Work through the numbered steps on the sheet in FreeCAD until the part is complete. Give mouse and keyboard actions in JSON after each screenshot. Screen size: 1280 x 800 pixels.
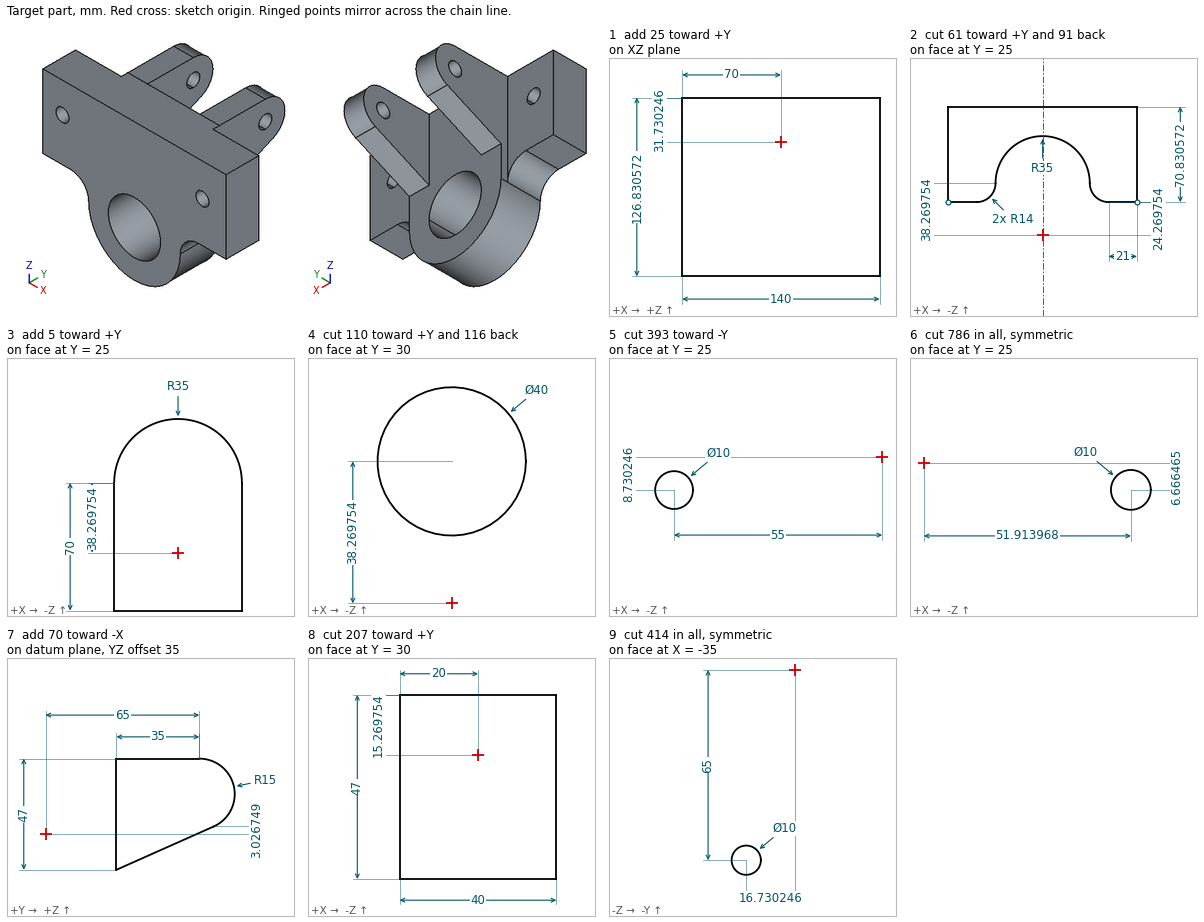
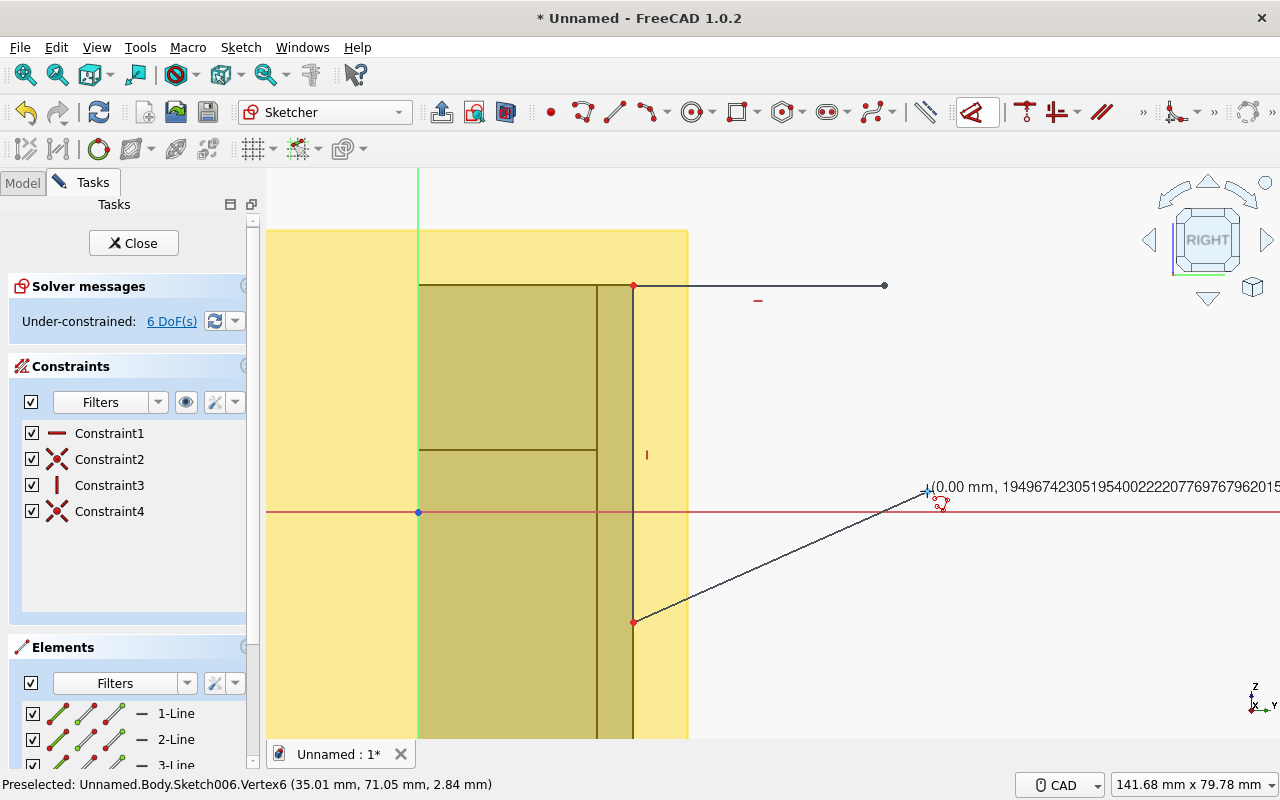
{"action": "left_click", "coordinate": [648, 112]}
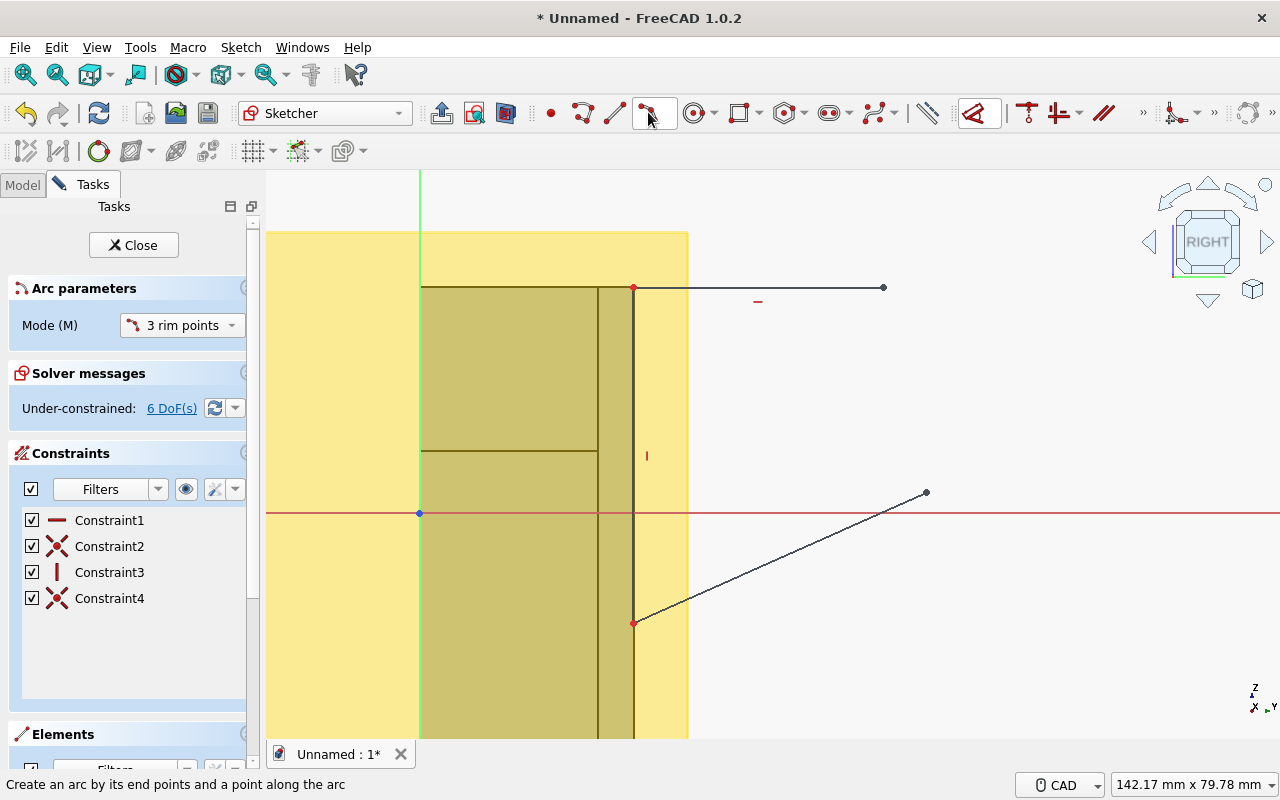
{"action": "left_click", "coordinate": [926, 493]}
{"action": "left_click", "coordinate": [884, 288]}
{"action": "left_click", "coordinate": [988, 372]}
{"action": "key", "text": "Escape"}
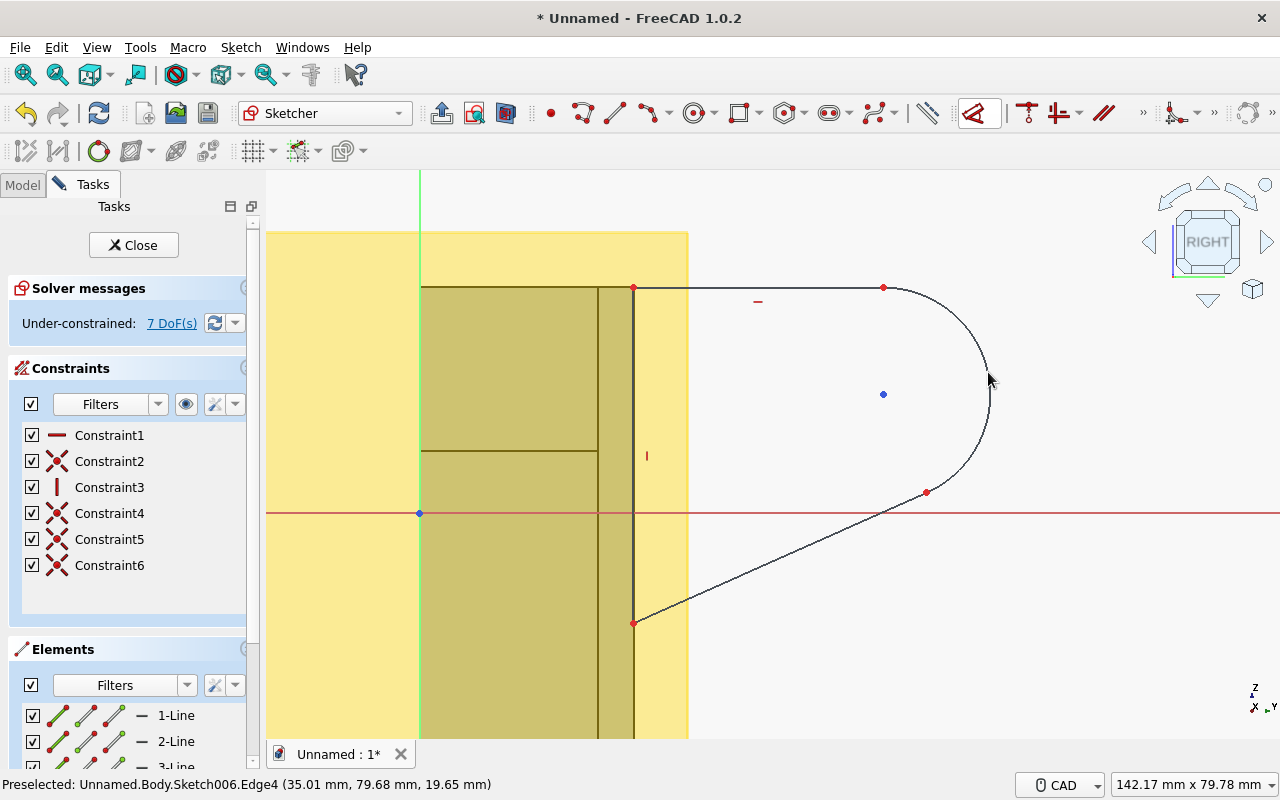
{"action": "left_click", "coordinate": [809, 288]}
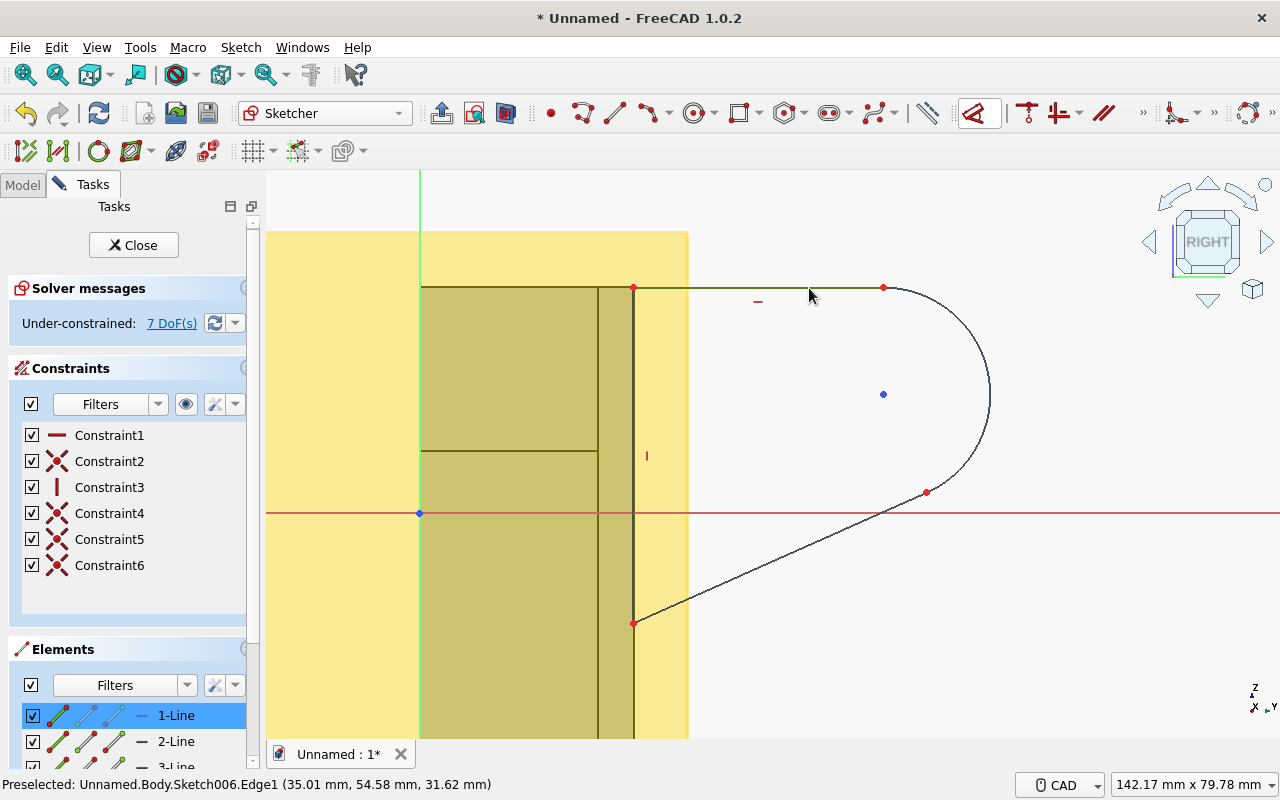
{"action": "left_click", "coordinate": [984, 430]}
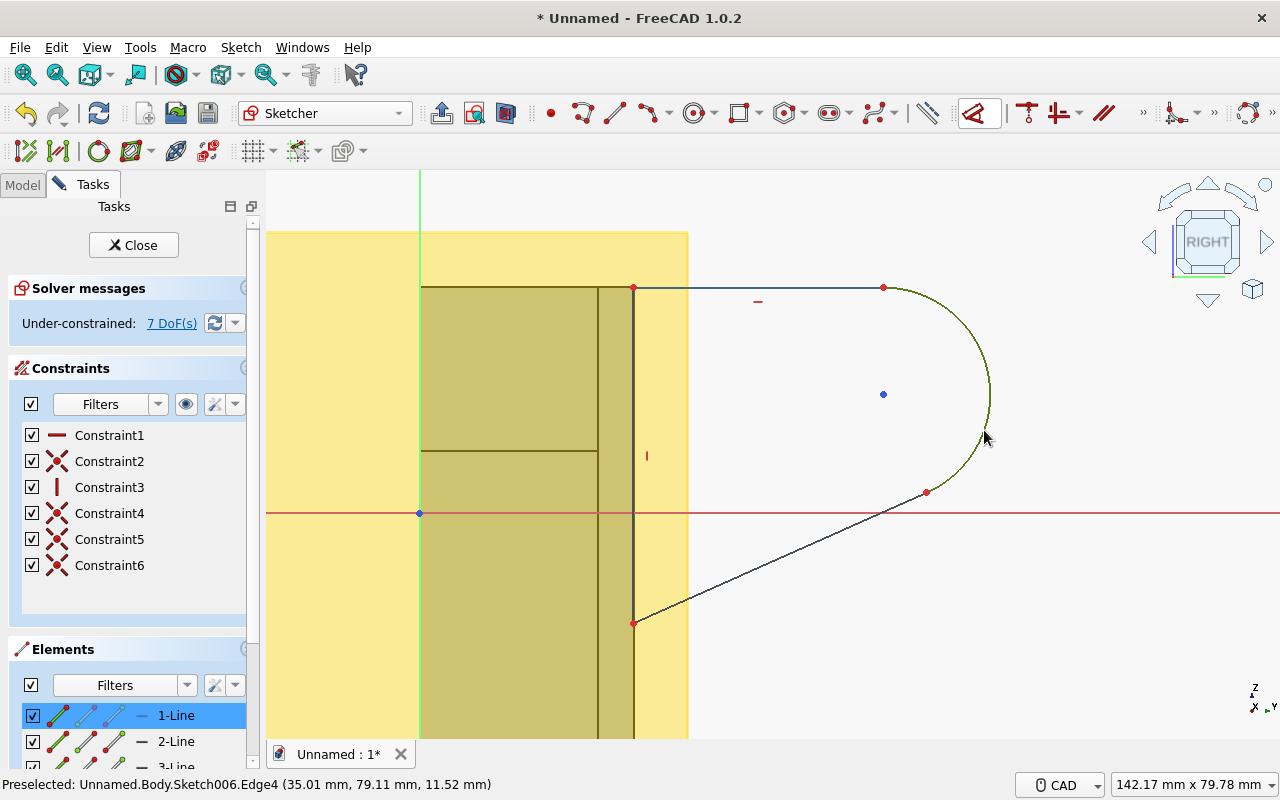
{"action": "key", "text": "t"}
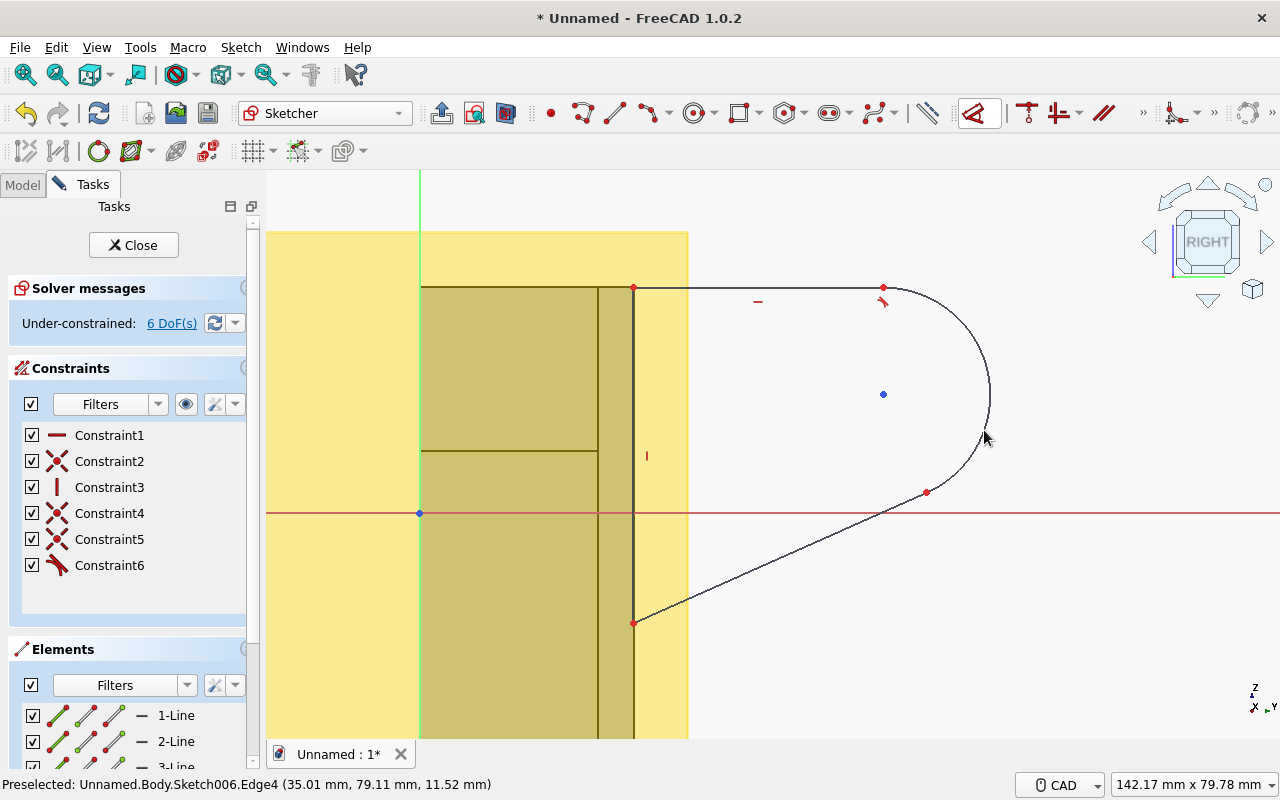
{"action": "left_click", "coordinate": [721, 584]}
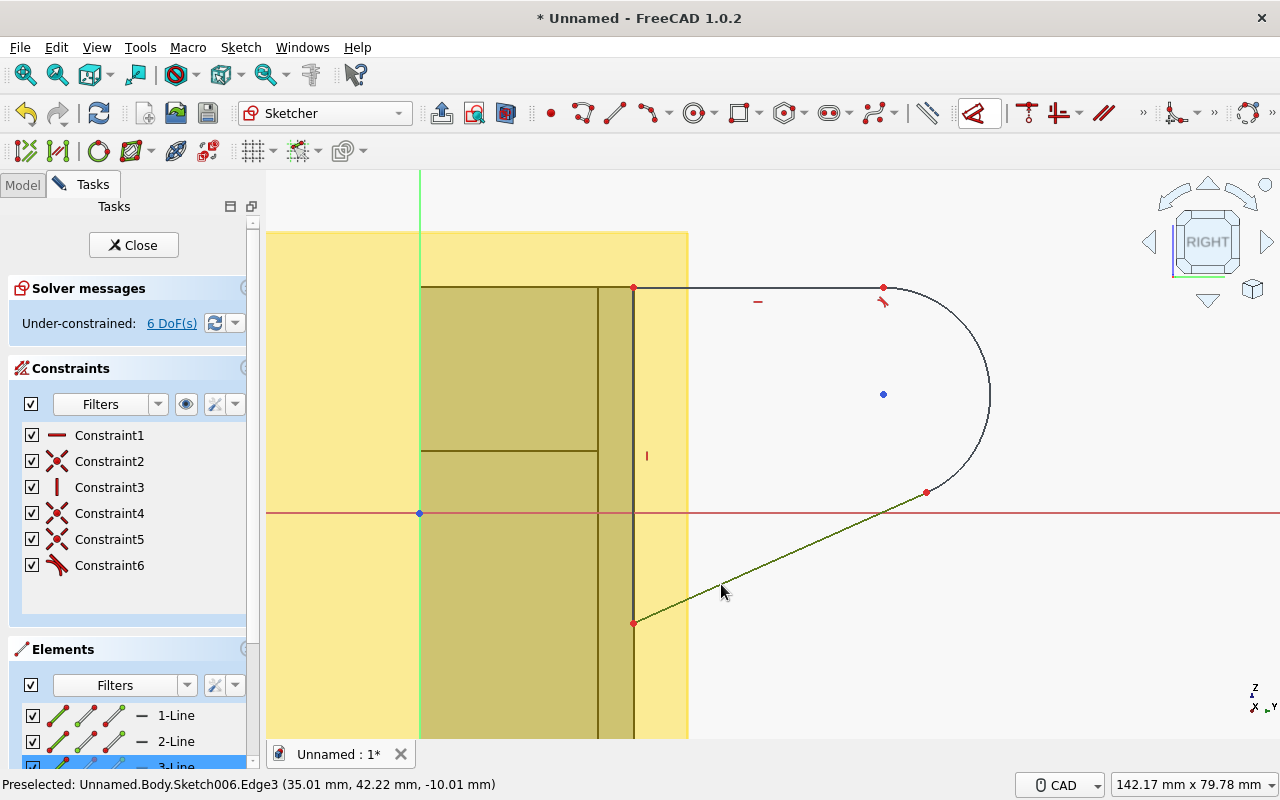
{"action": "left_click", "coordinate": [984, 430]}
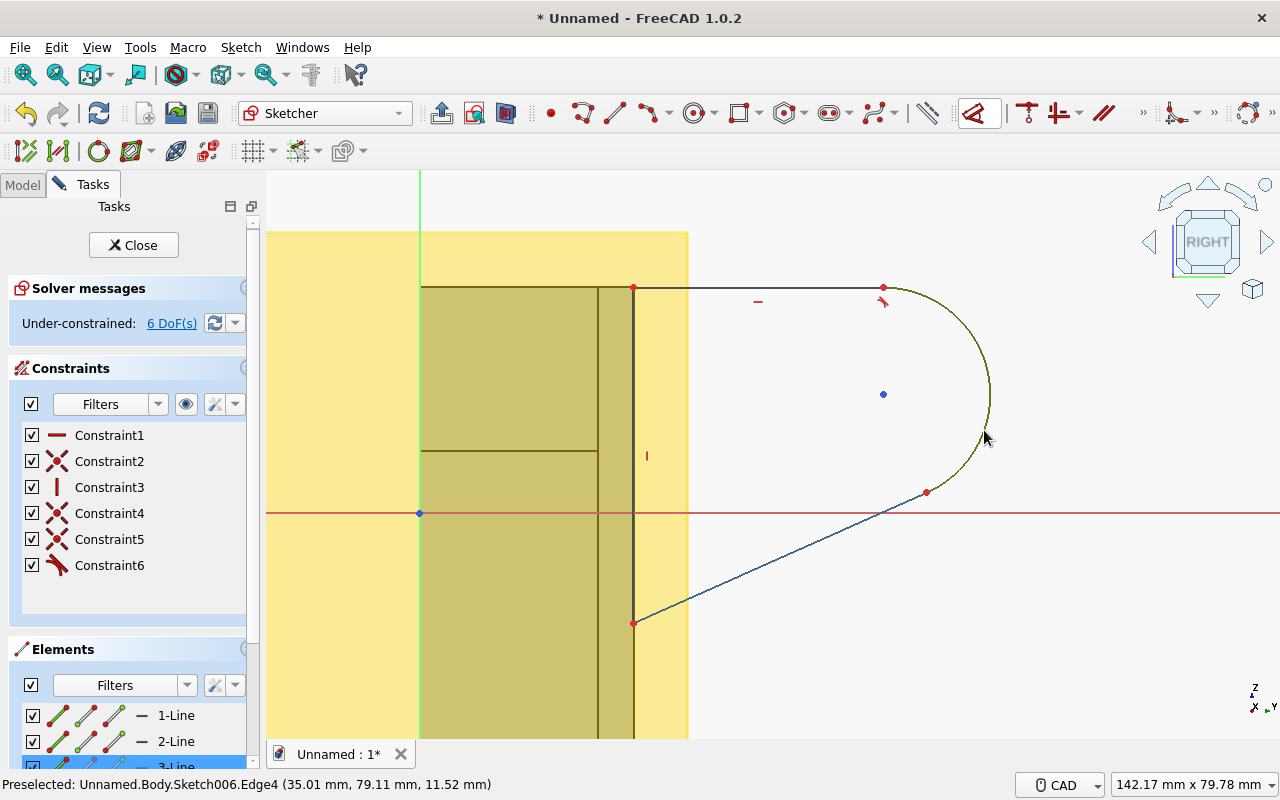
{"action": "key", "text": "t"}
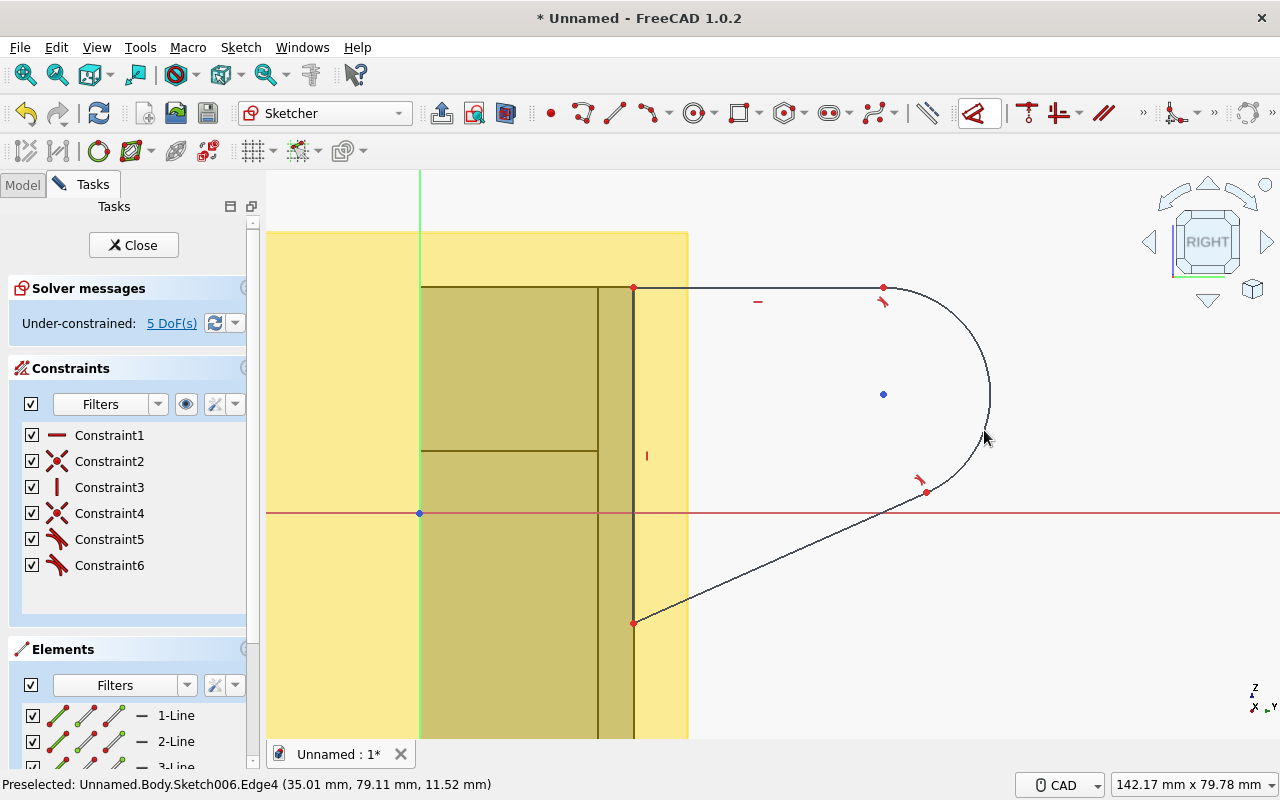
{"action": "left_click", "coordinate": [984, 430]}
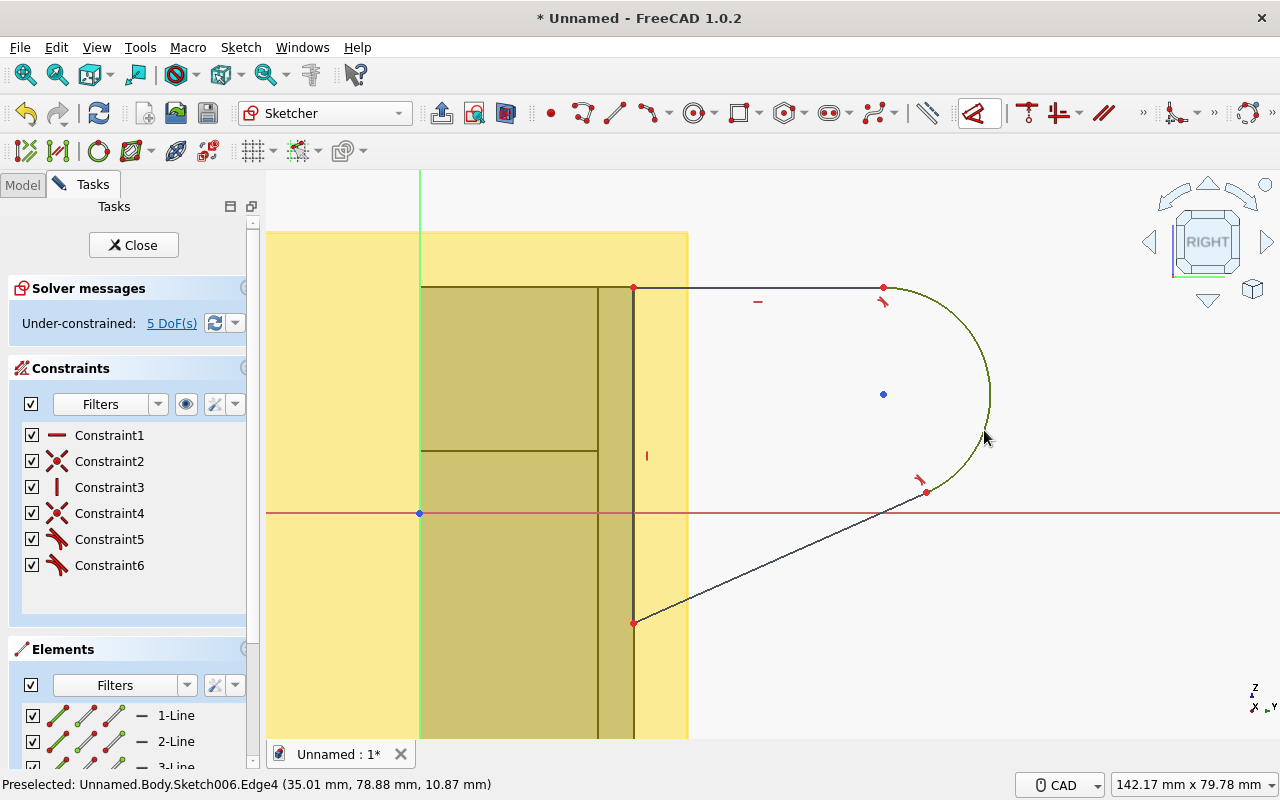
{"action": "left_click", "coordinate": [996, 114]}